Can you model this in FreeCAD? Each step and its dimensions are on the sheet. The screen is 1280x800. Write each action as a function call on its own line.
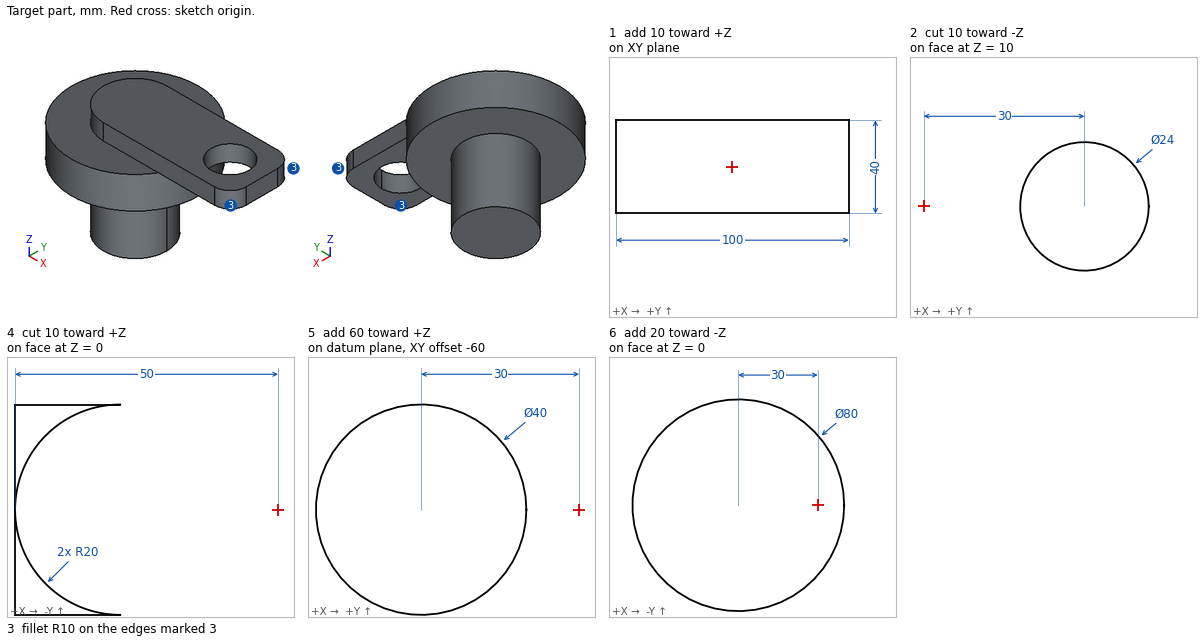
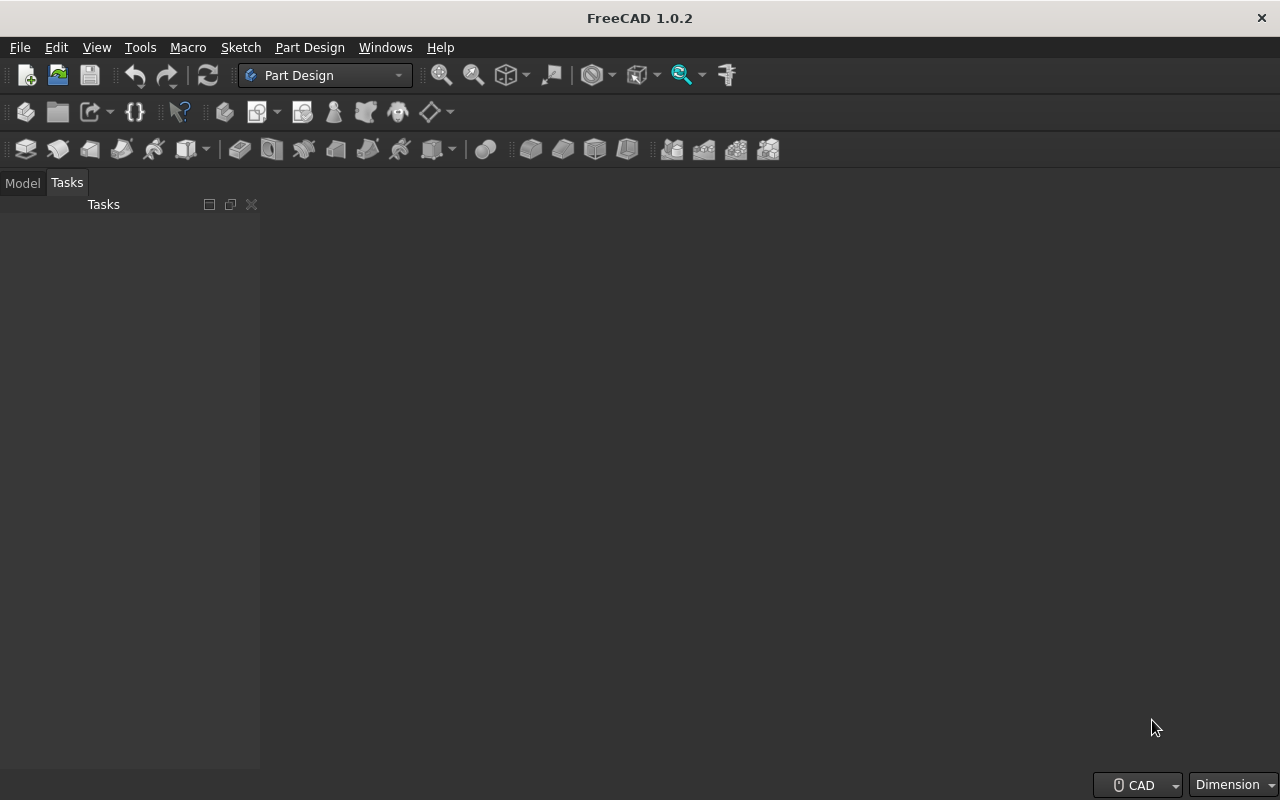
click(26, 76)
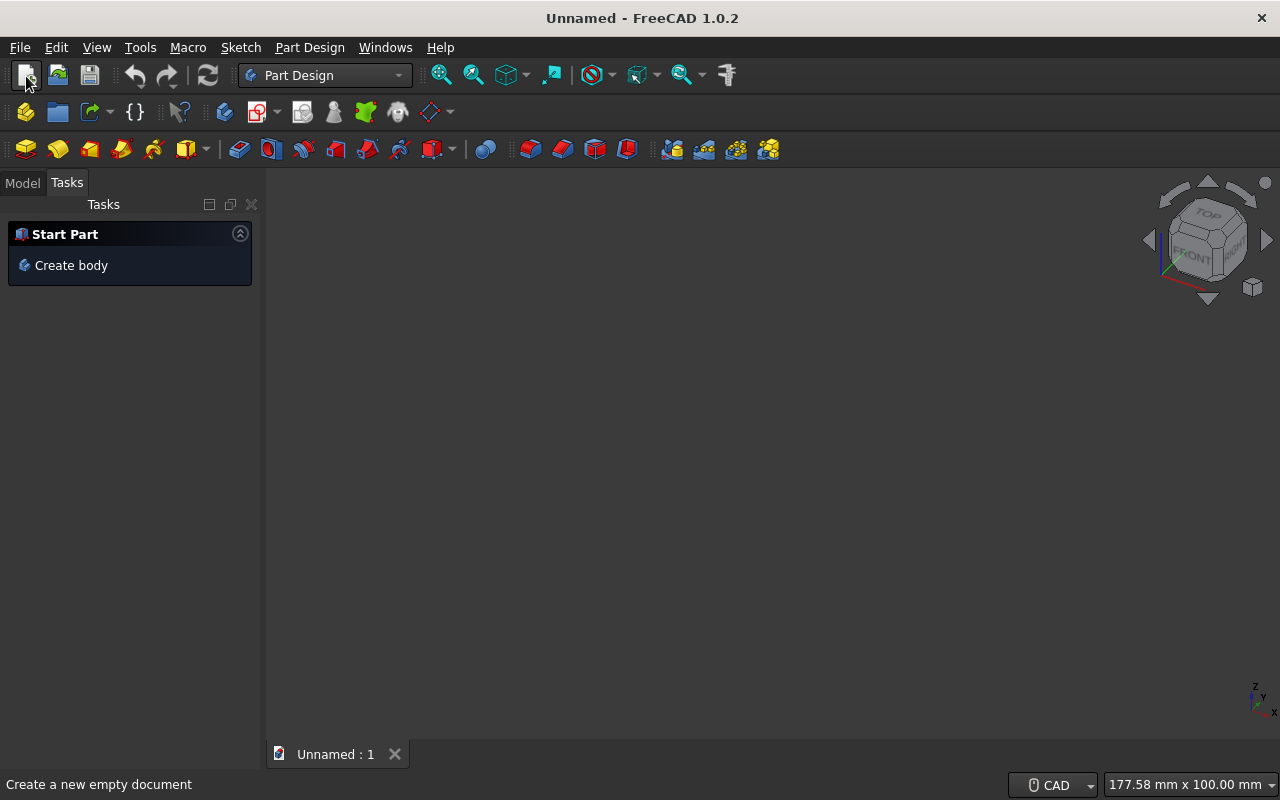
click(258, 112)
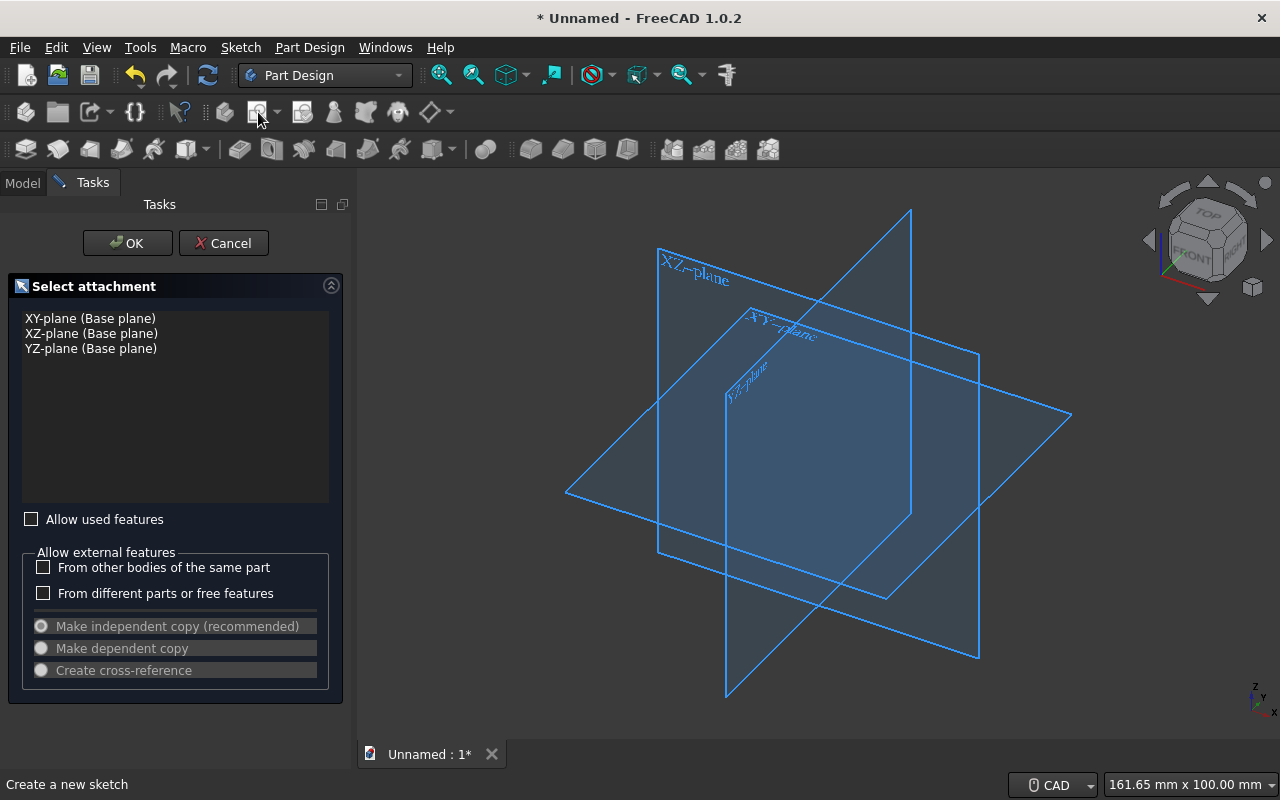
click(82, 318)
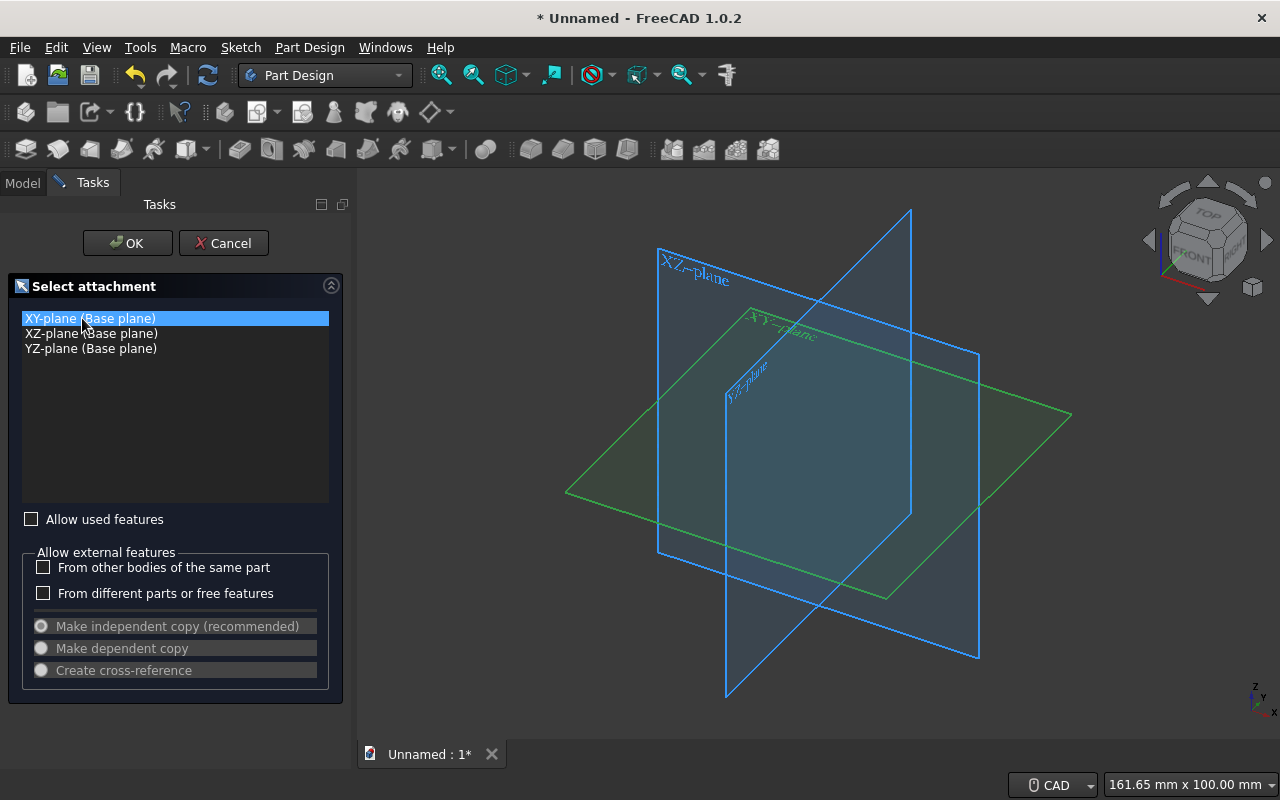
click(128, 243)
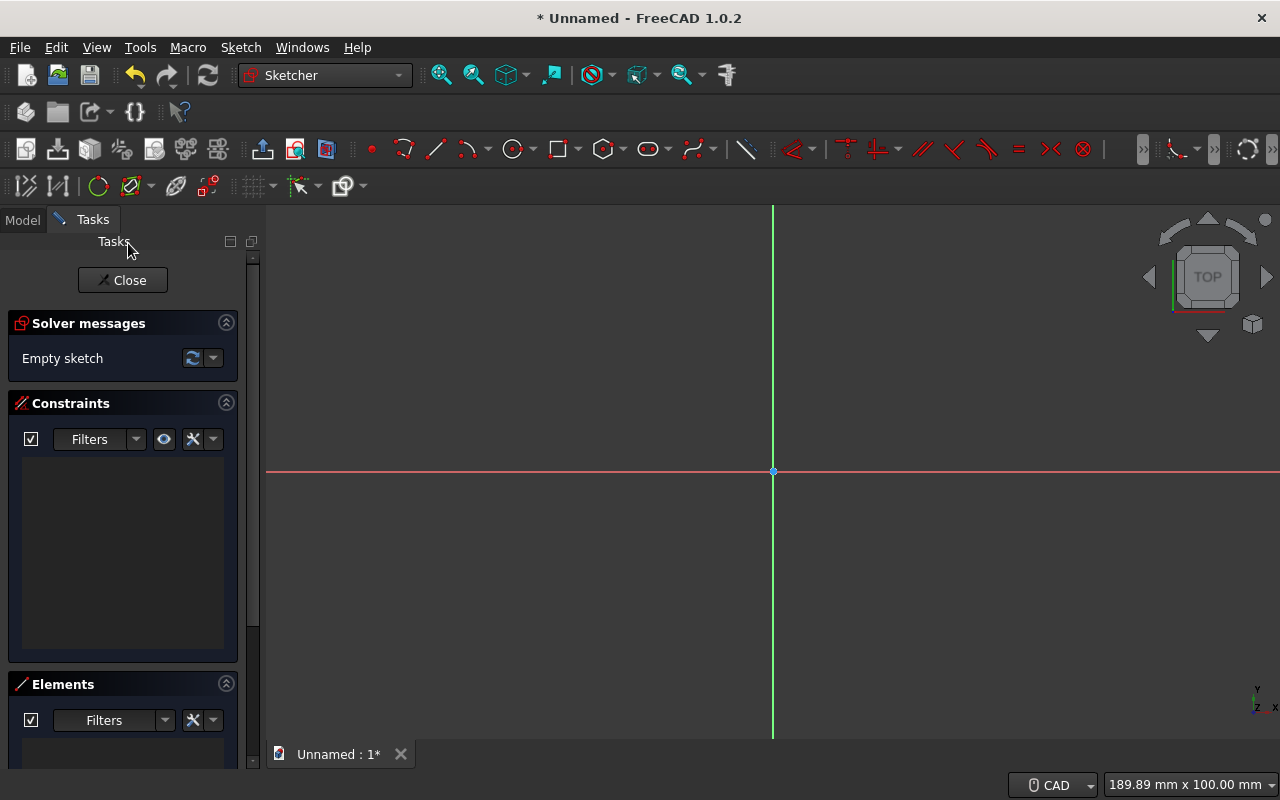
key(g)
key(v)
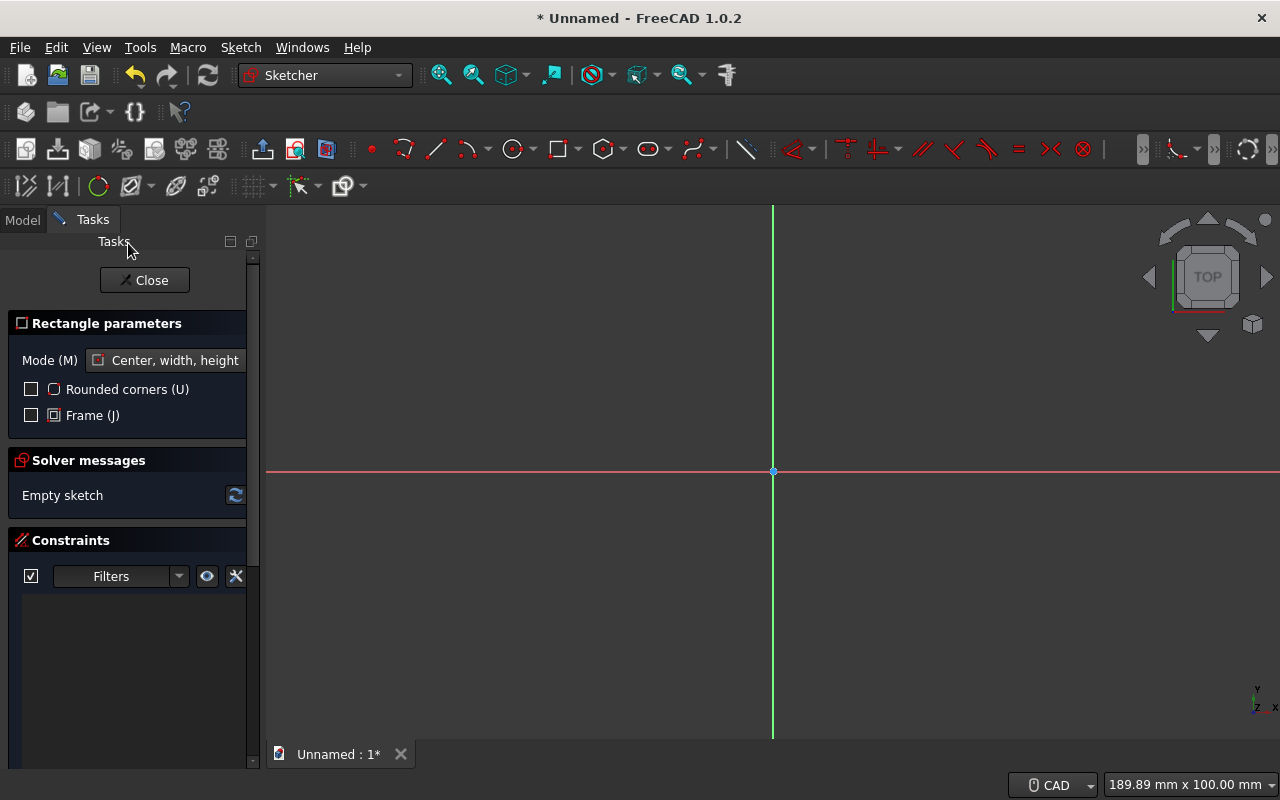
click(773, 472)
move(1040, 365)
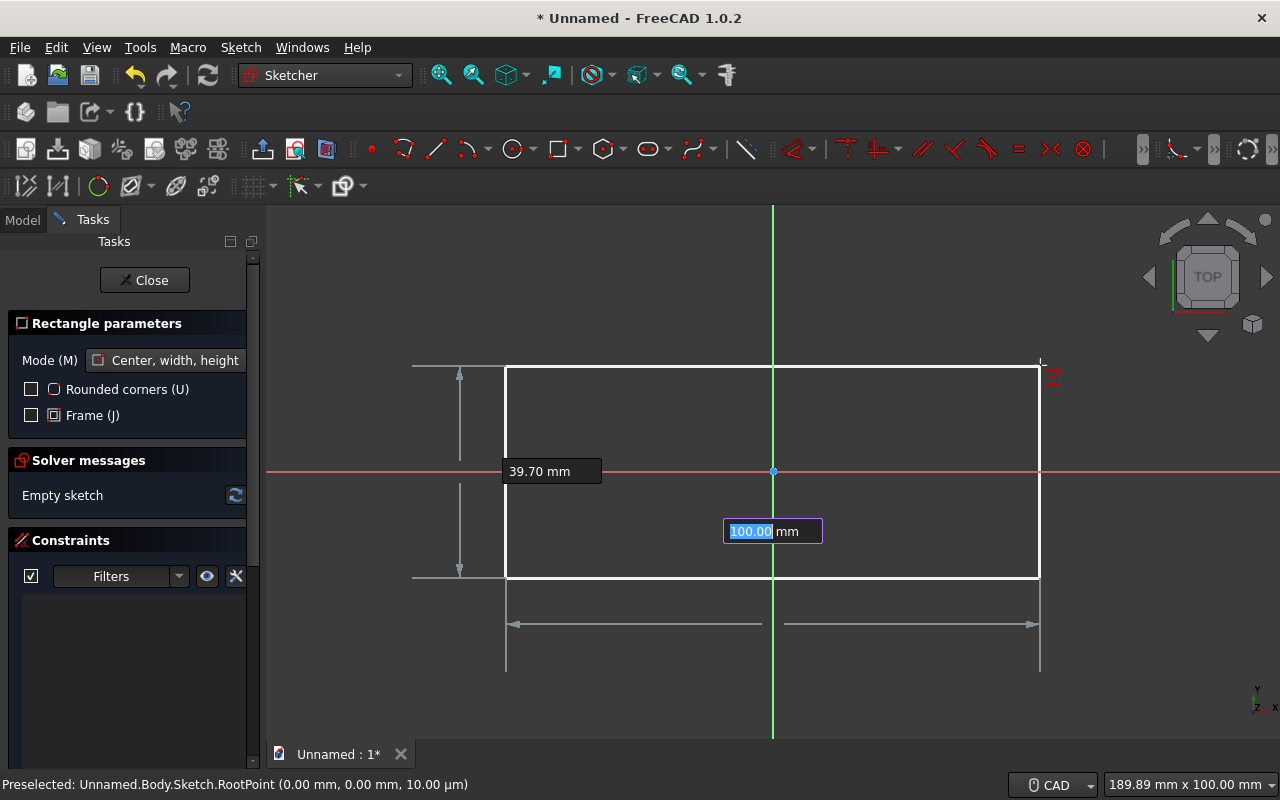
text(100)
key(Tab)
text(40)
key(Return)
key(Escape)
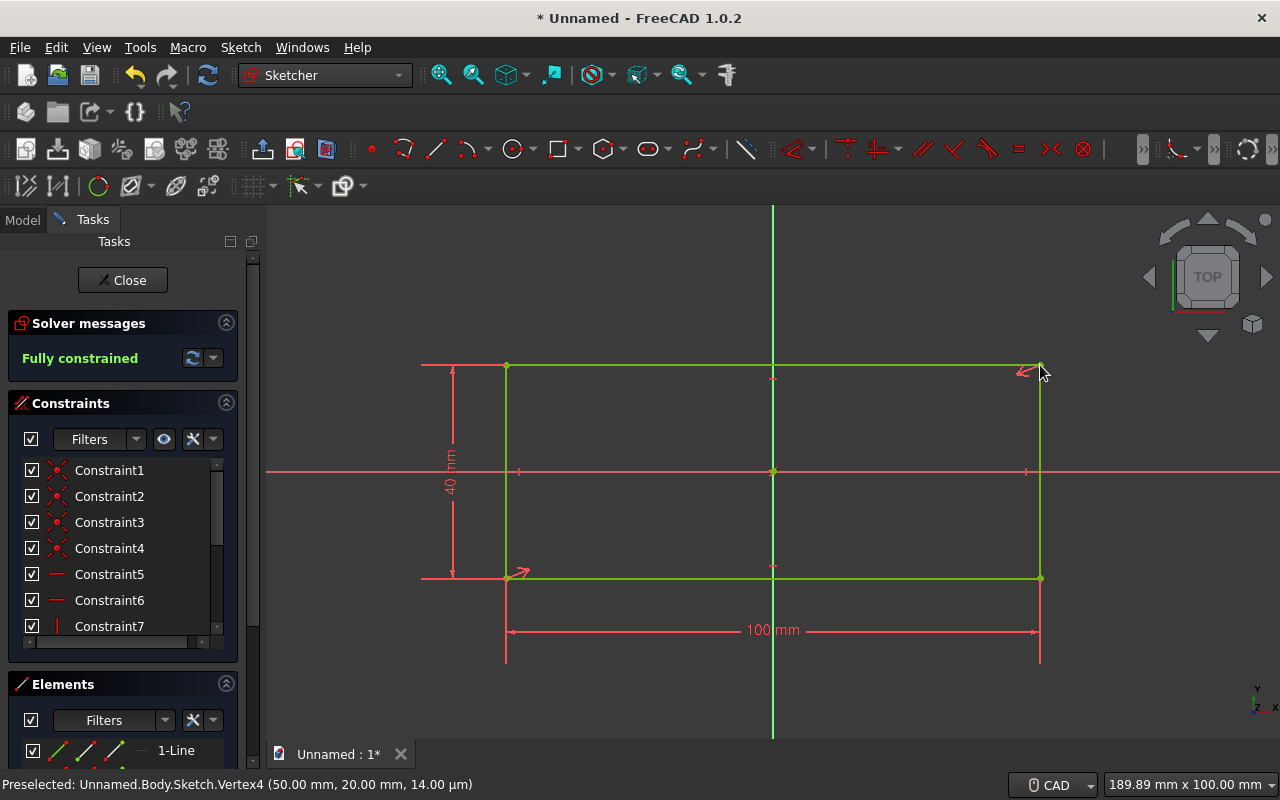
click(123, 280)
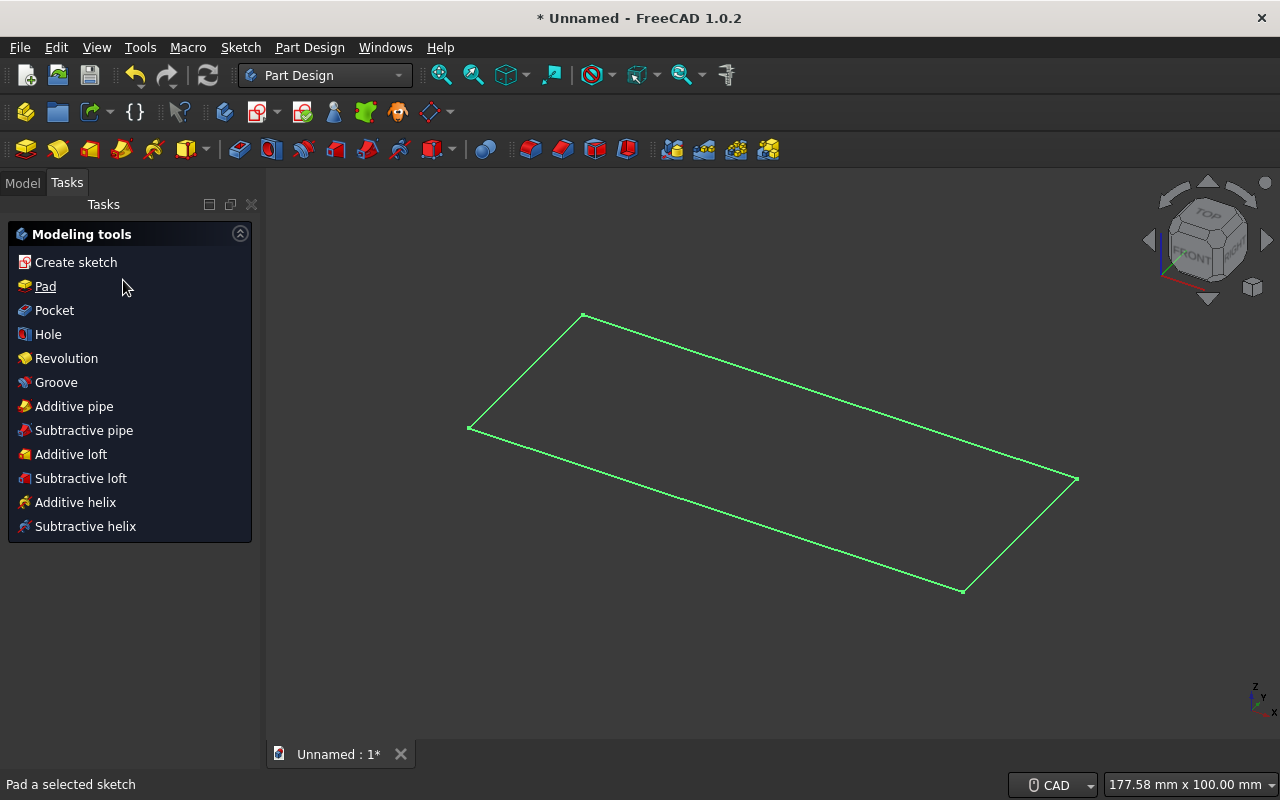
click(26, 150)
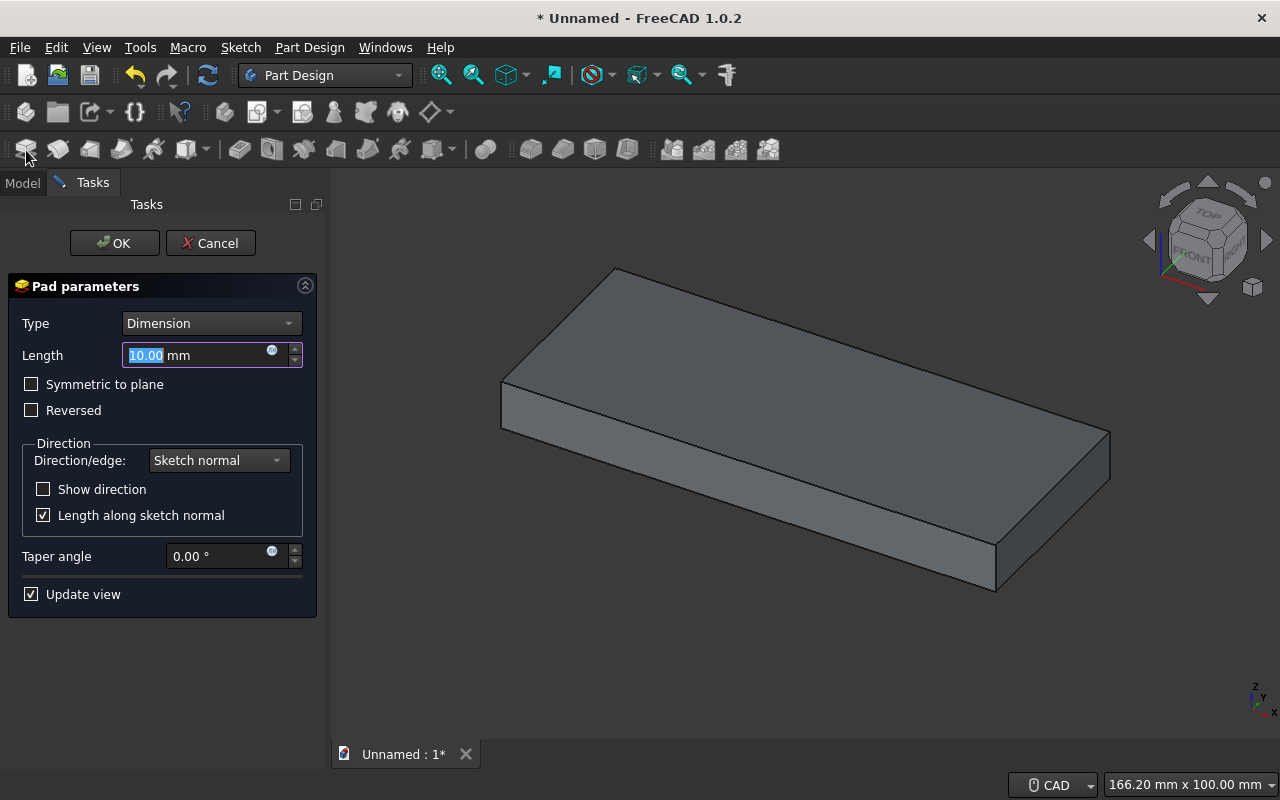
text(10)
key(Tab)